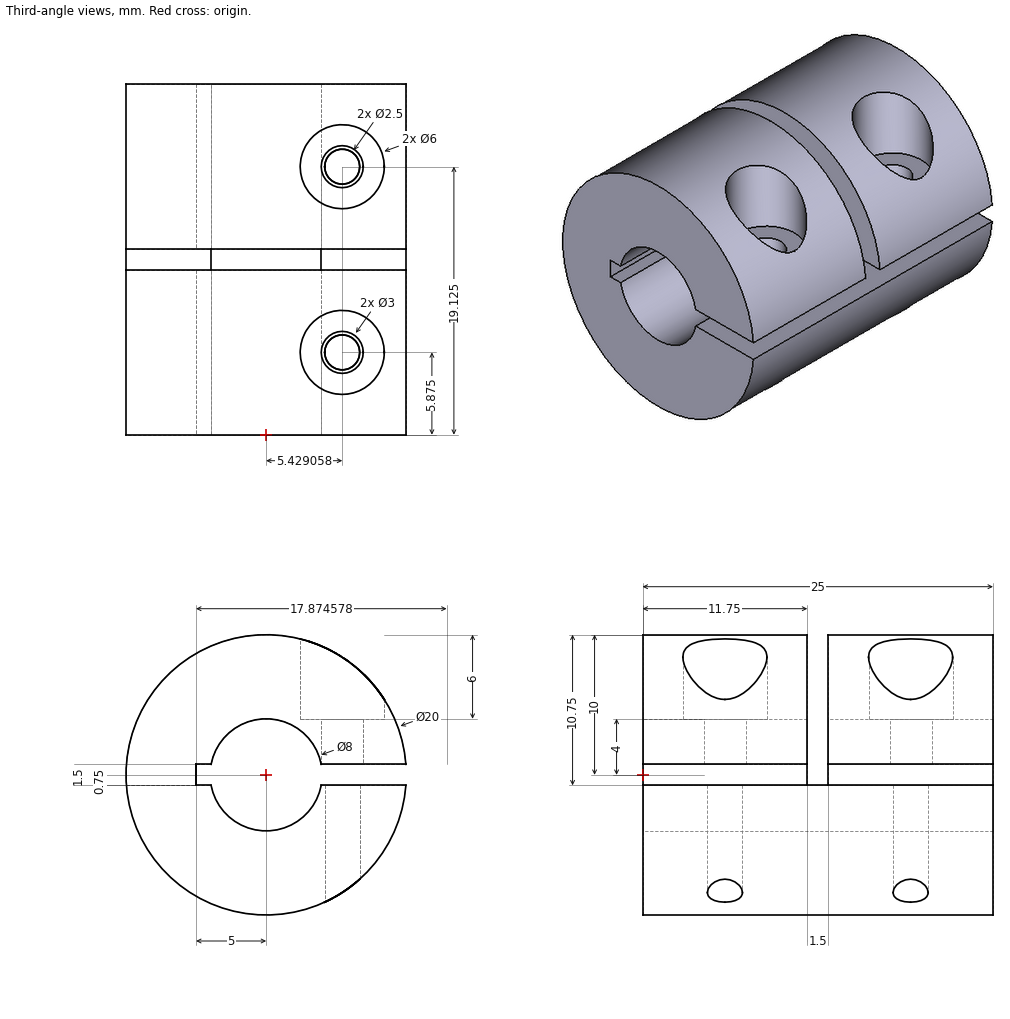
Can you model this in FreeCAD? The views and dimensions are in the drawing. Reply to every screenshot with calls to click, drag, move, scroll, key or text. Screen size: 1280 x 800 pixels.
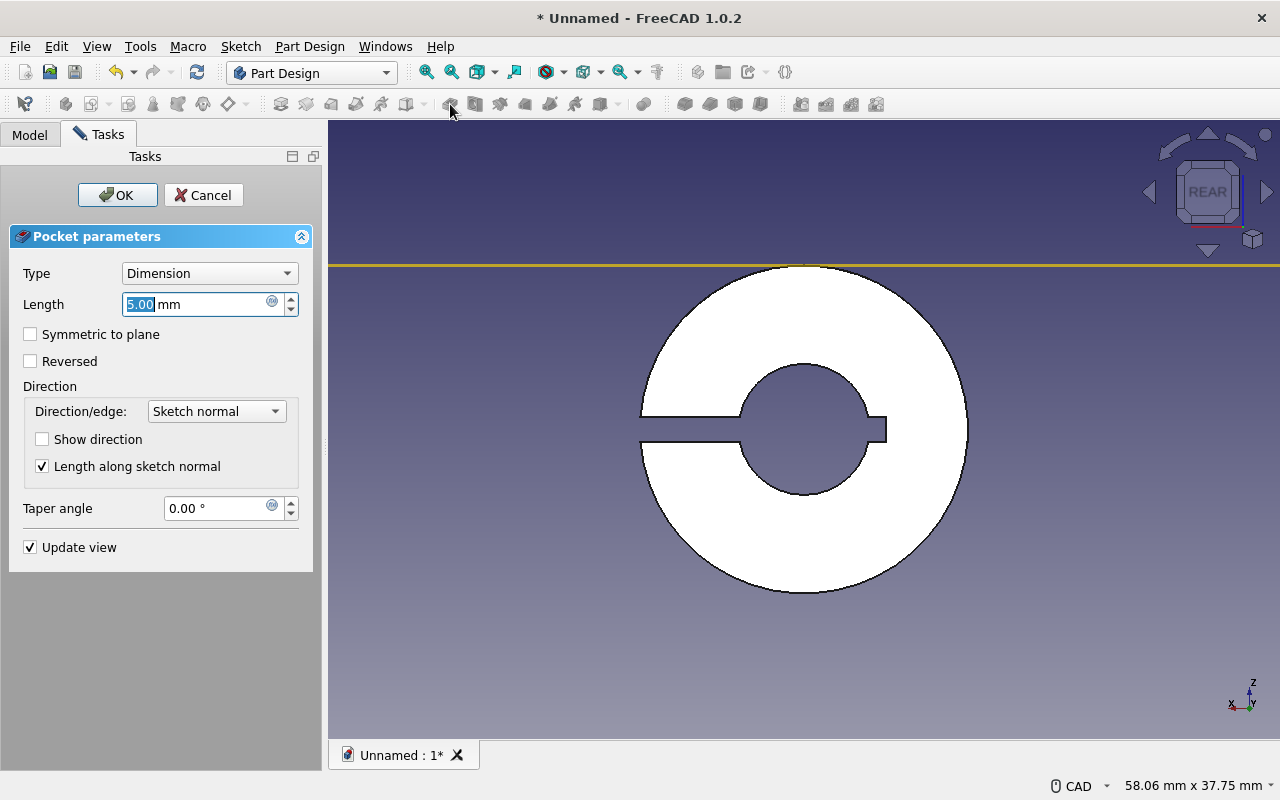
text(6)
key(Tab)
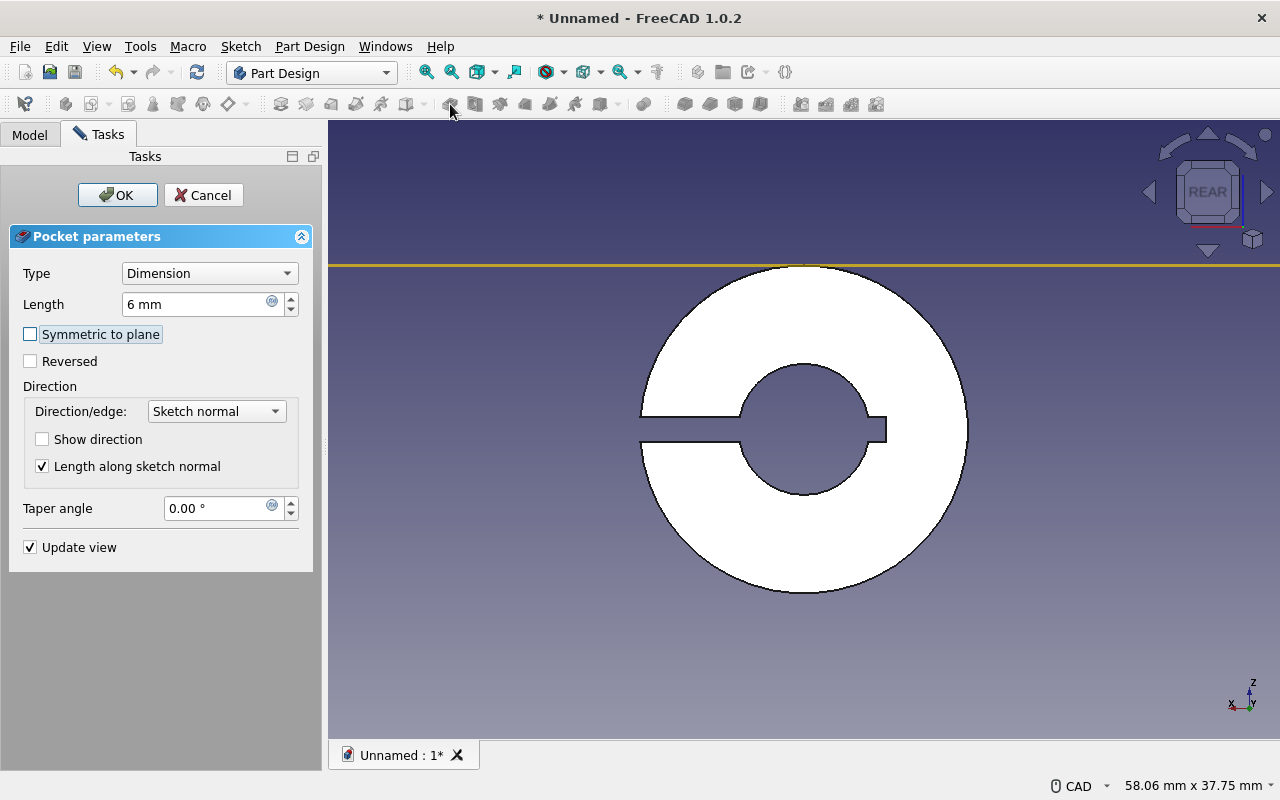
click(118, 195)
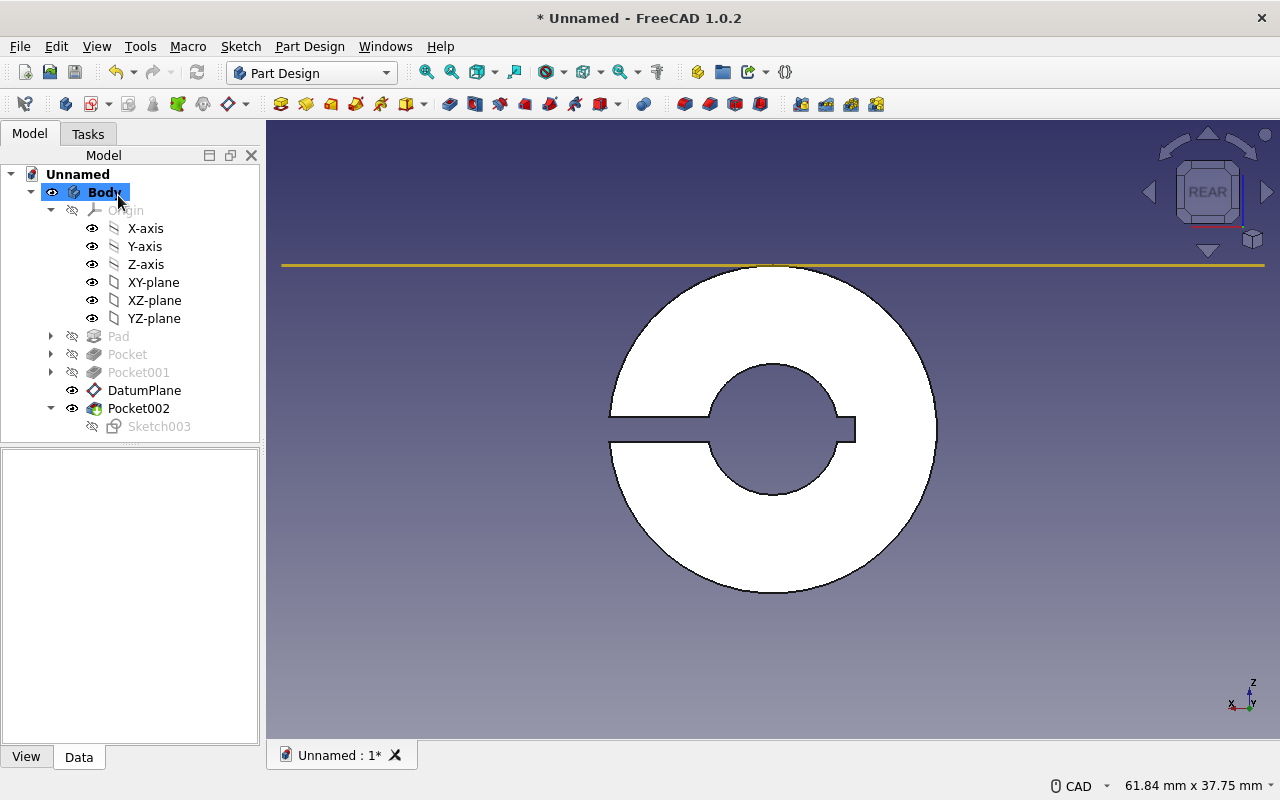
click(117, 390)
key(space)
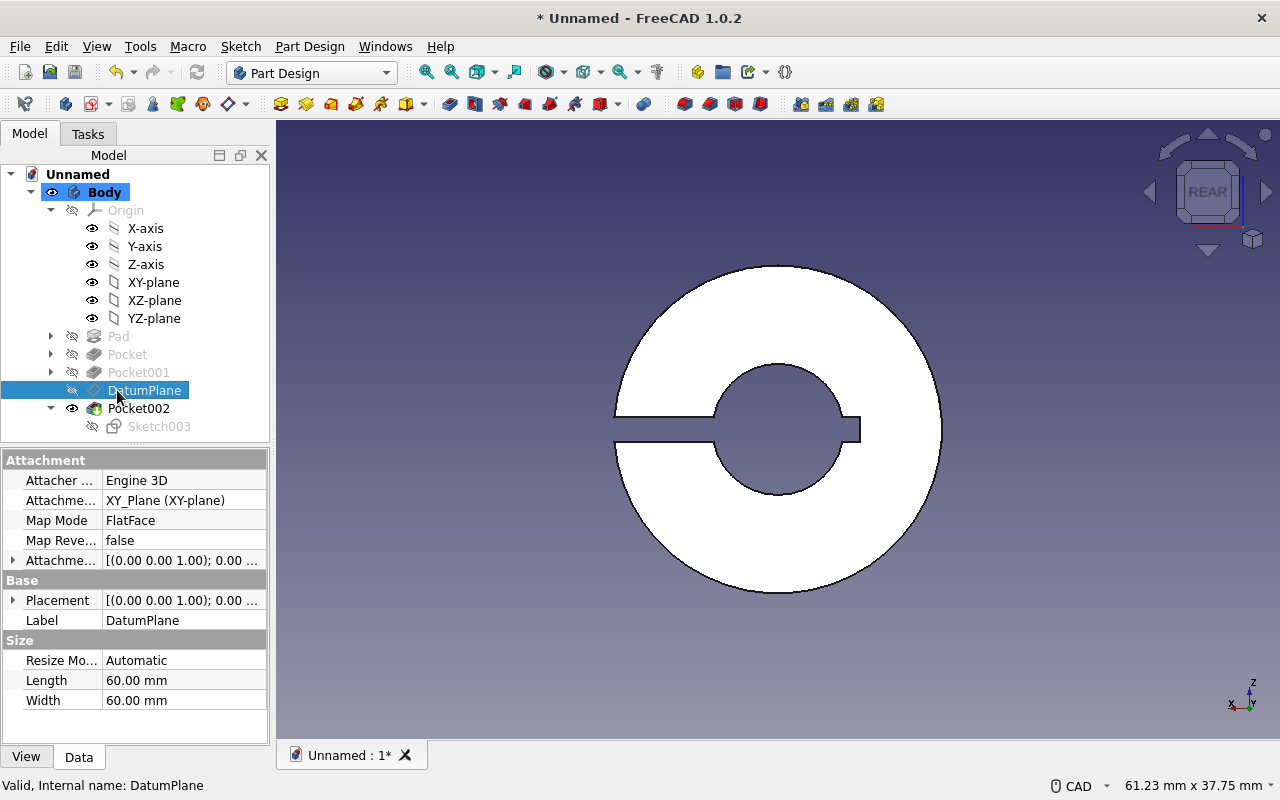
key(0)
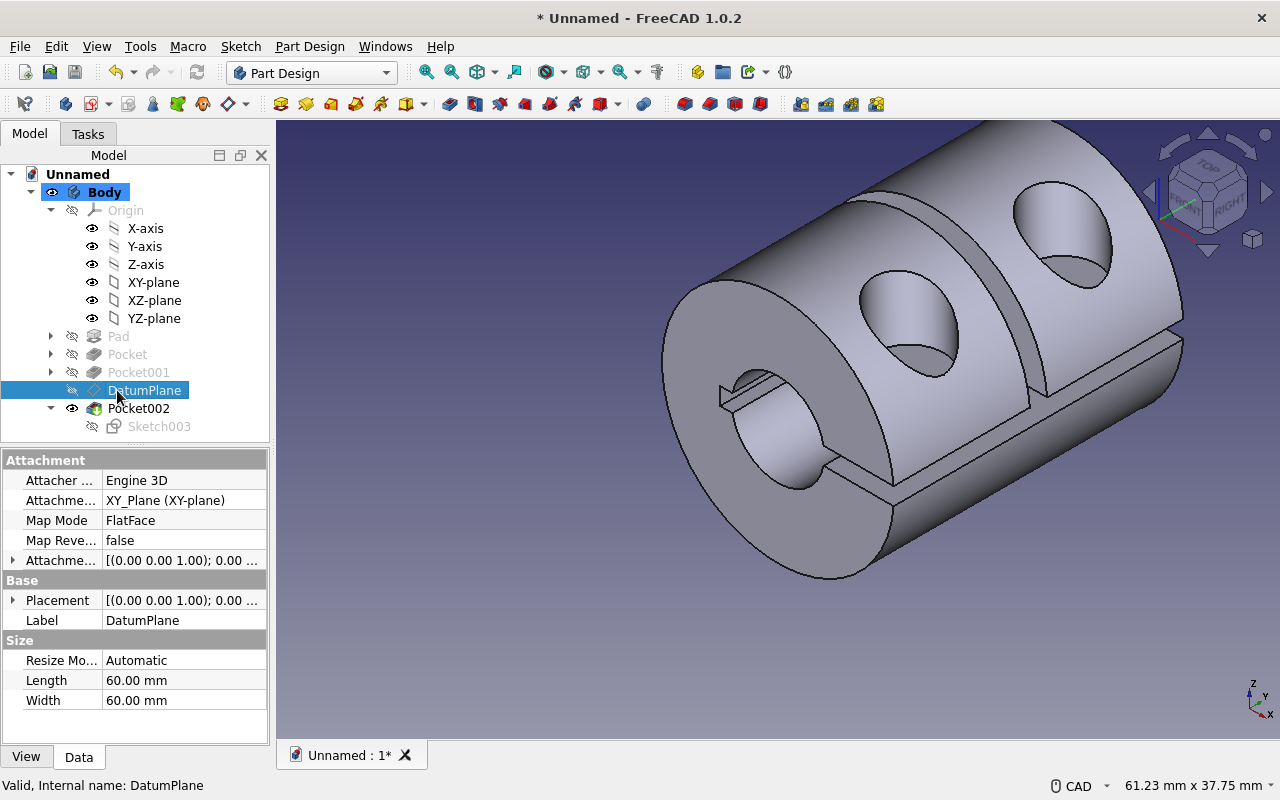
click(427, 72)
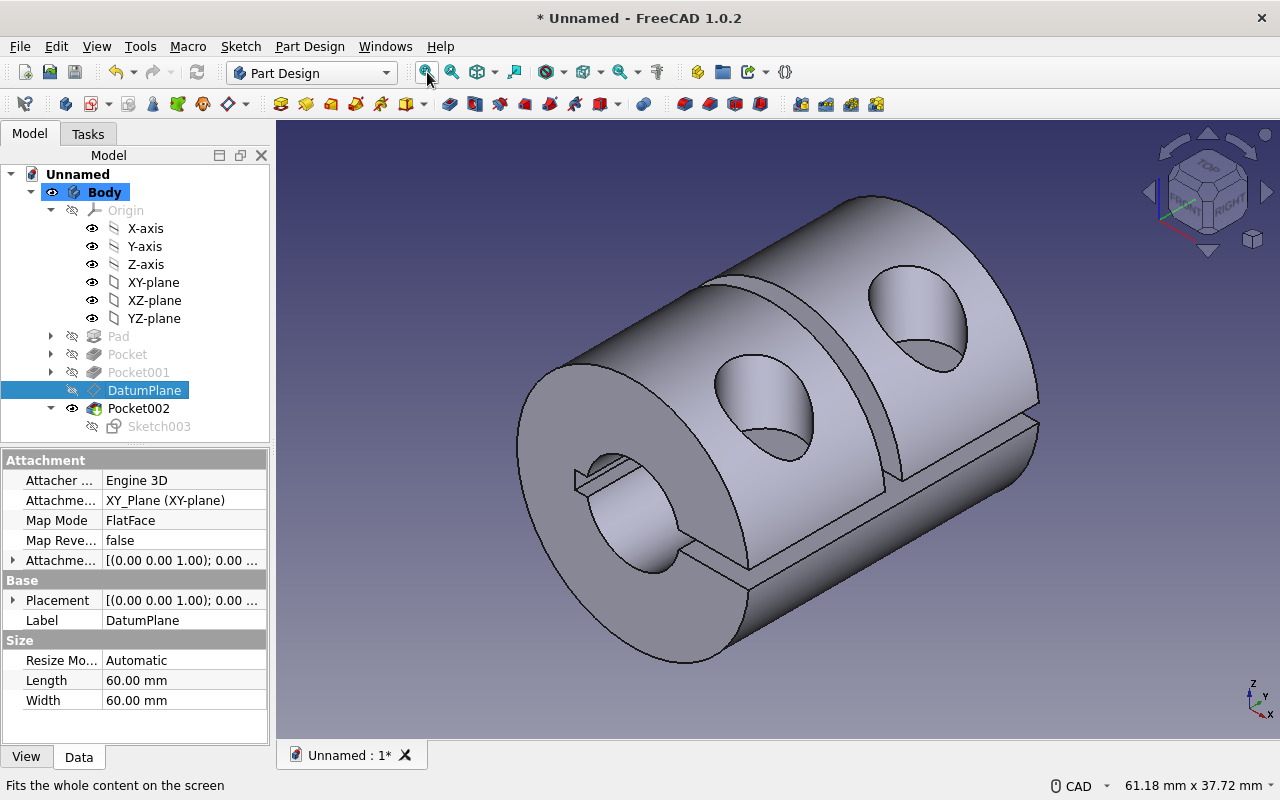
key(2)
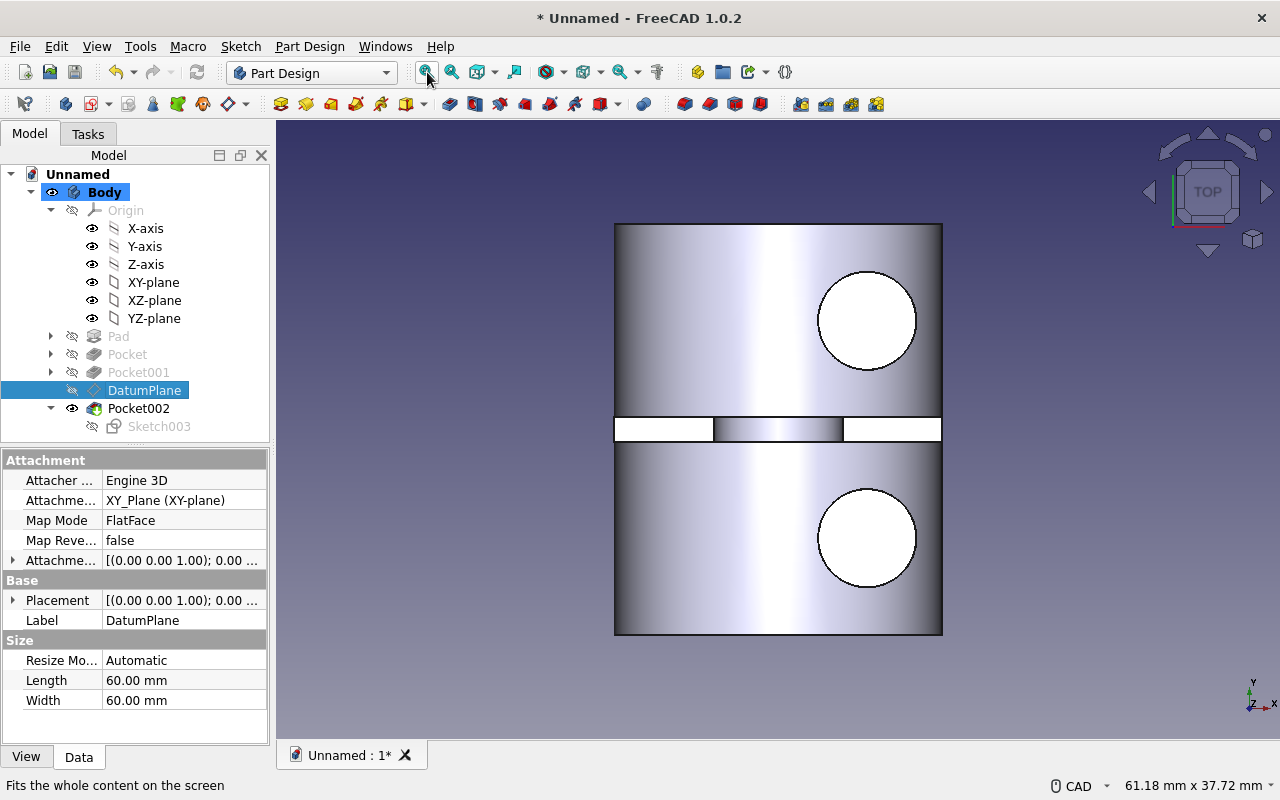
click(867, 537)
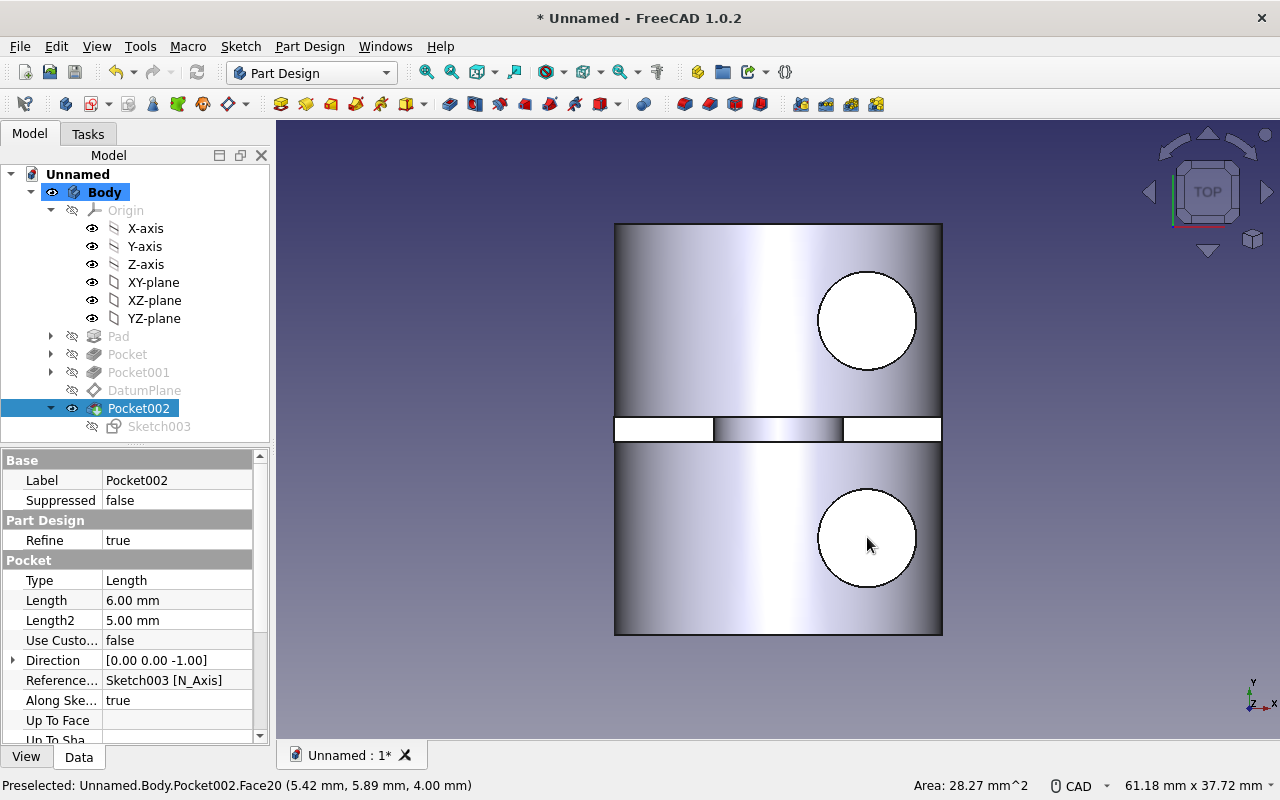
click(90, 104)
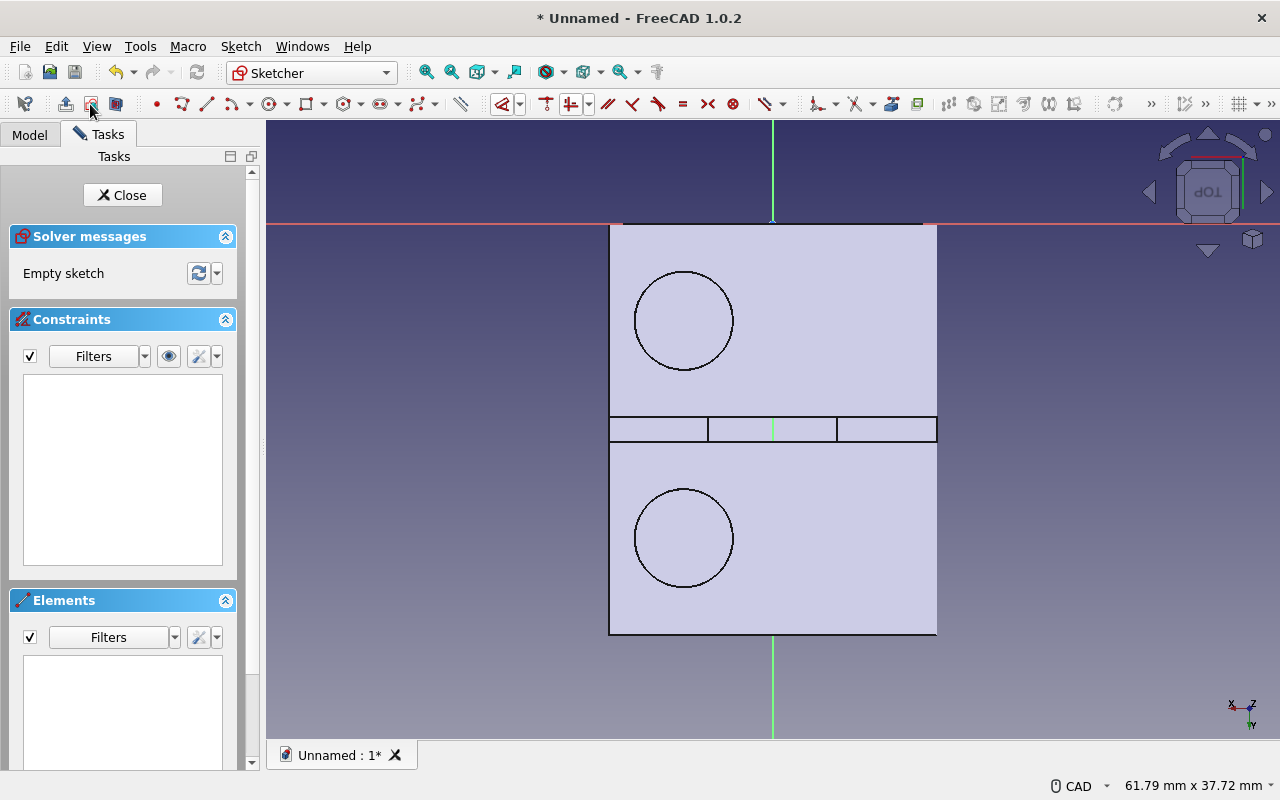
click(116, 104)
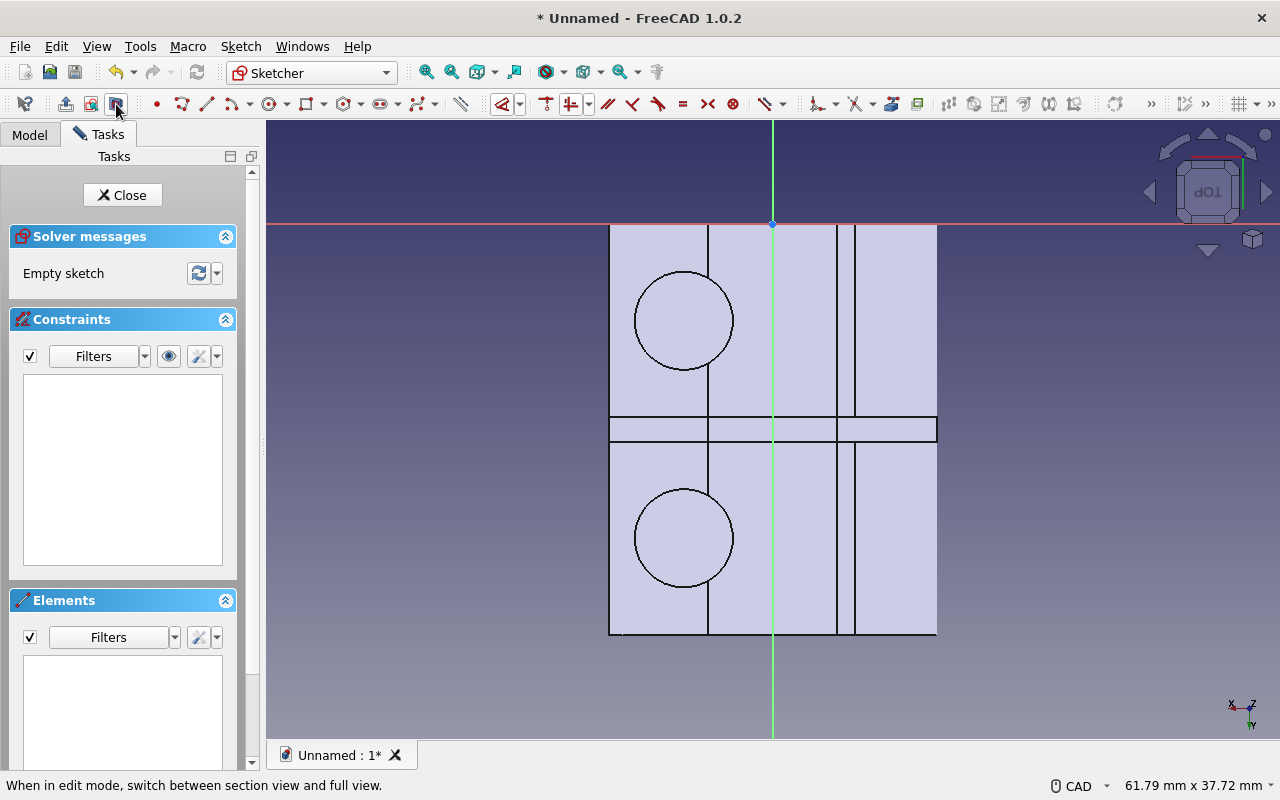
click(268, 104)